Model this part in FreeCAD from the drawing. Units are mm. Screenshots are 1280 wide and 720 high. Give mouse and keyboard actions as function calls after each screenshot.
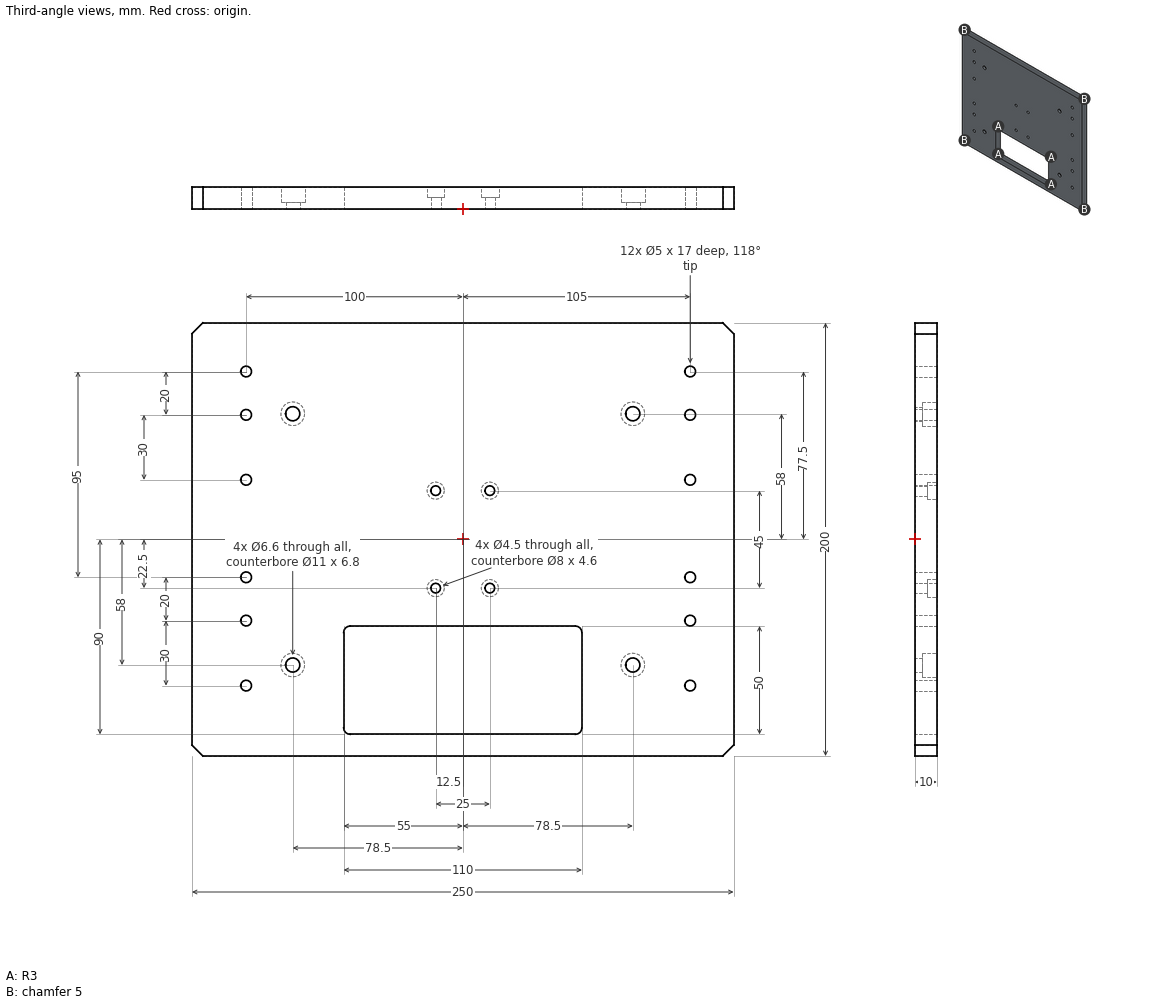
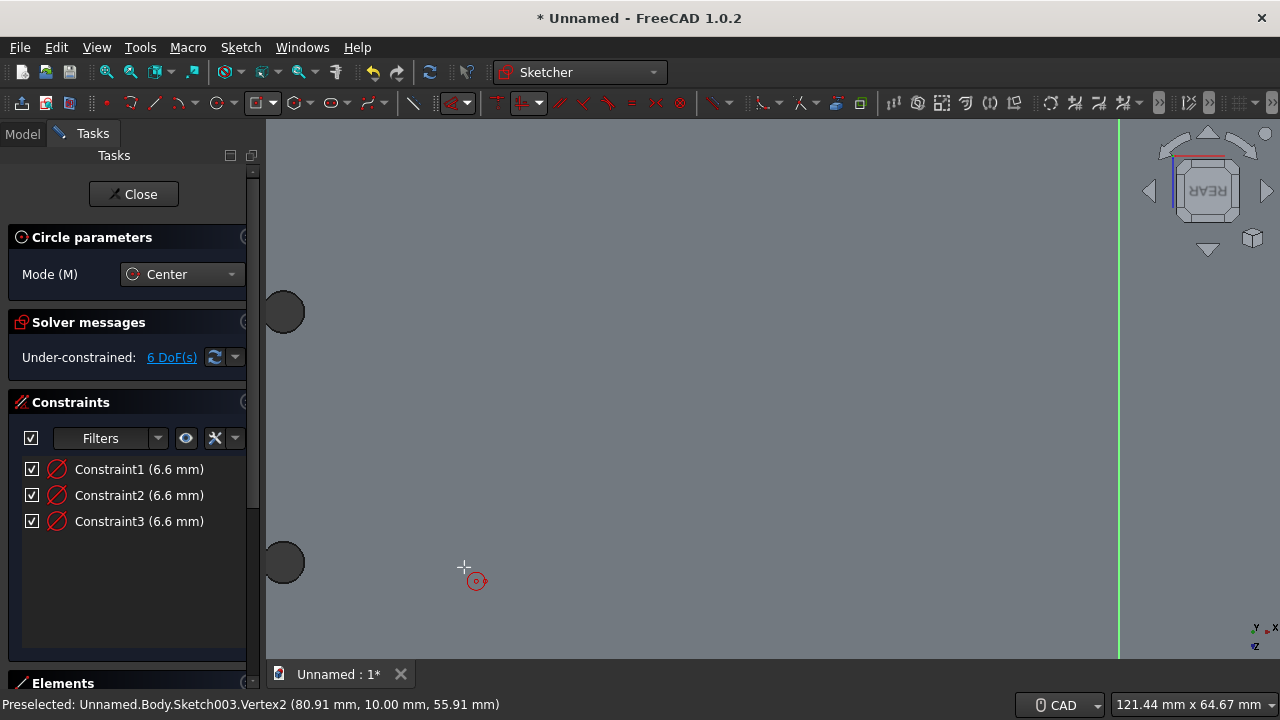
click(463, 567)
move(483, 547)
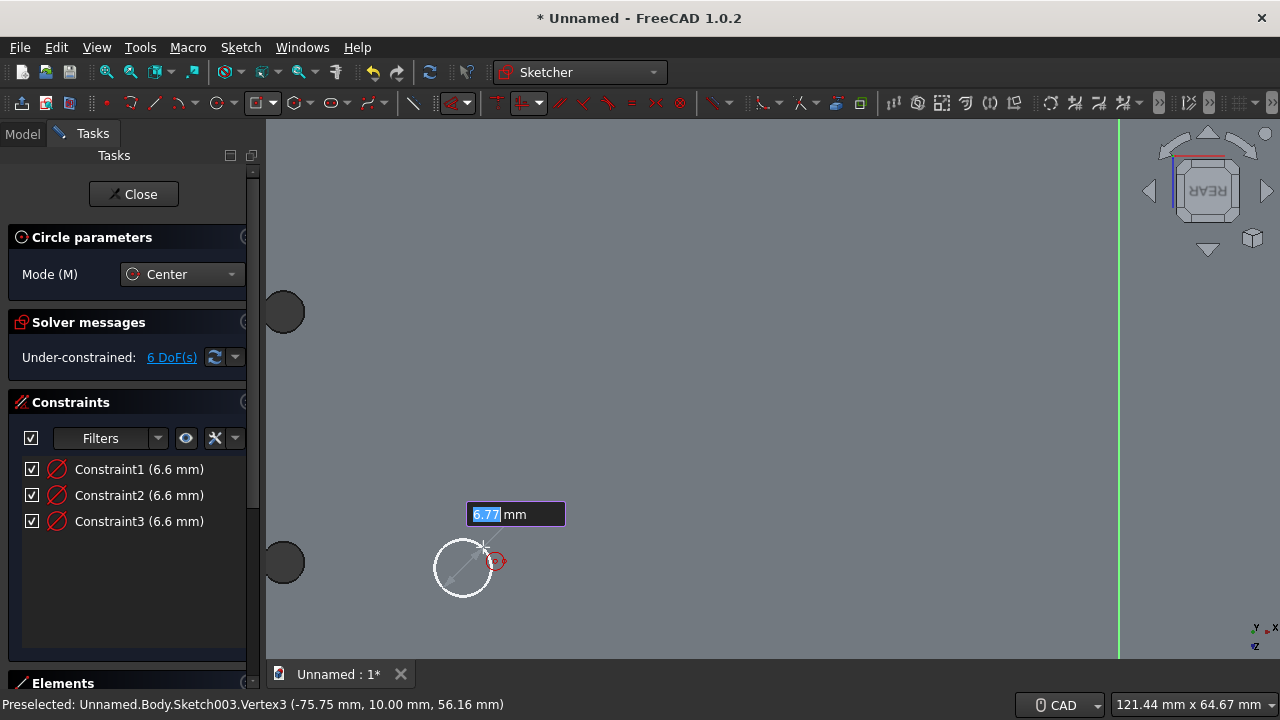
text(6.6)
key(Return)
key(Escape)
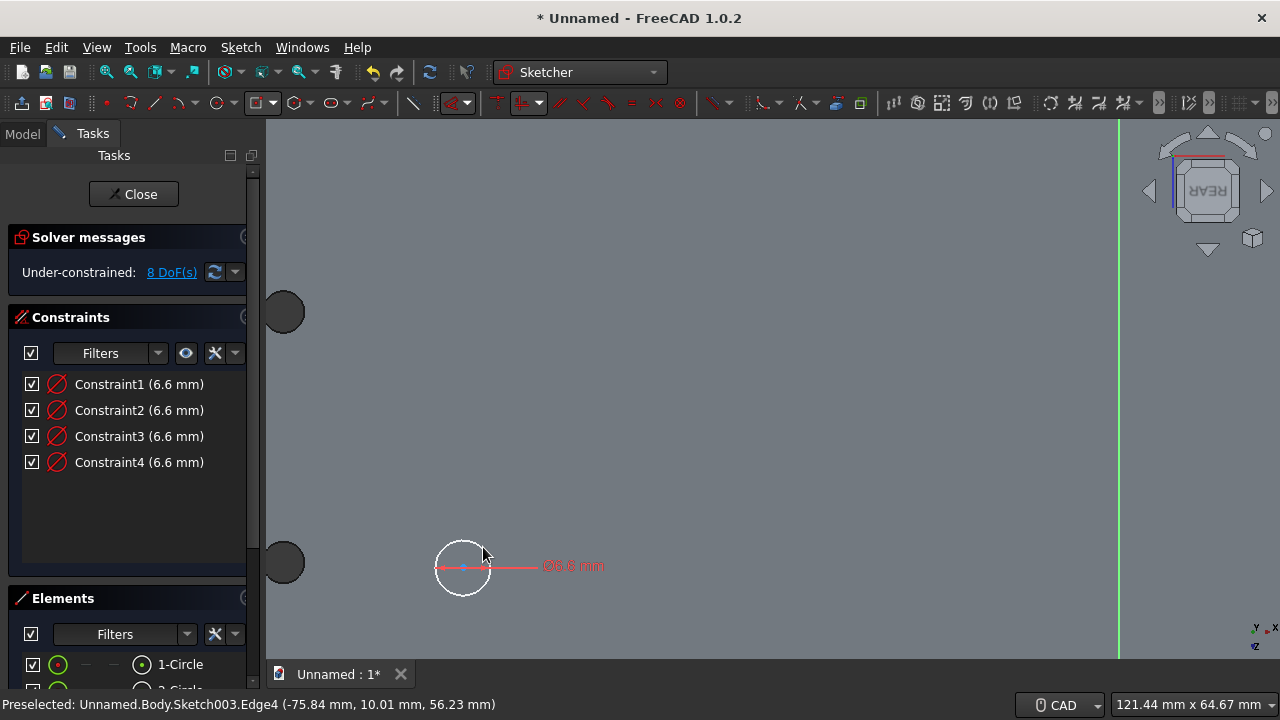
scroll(464, 567, down, 5)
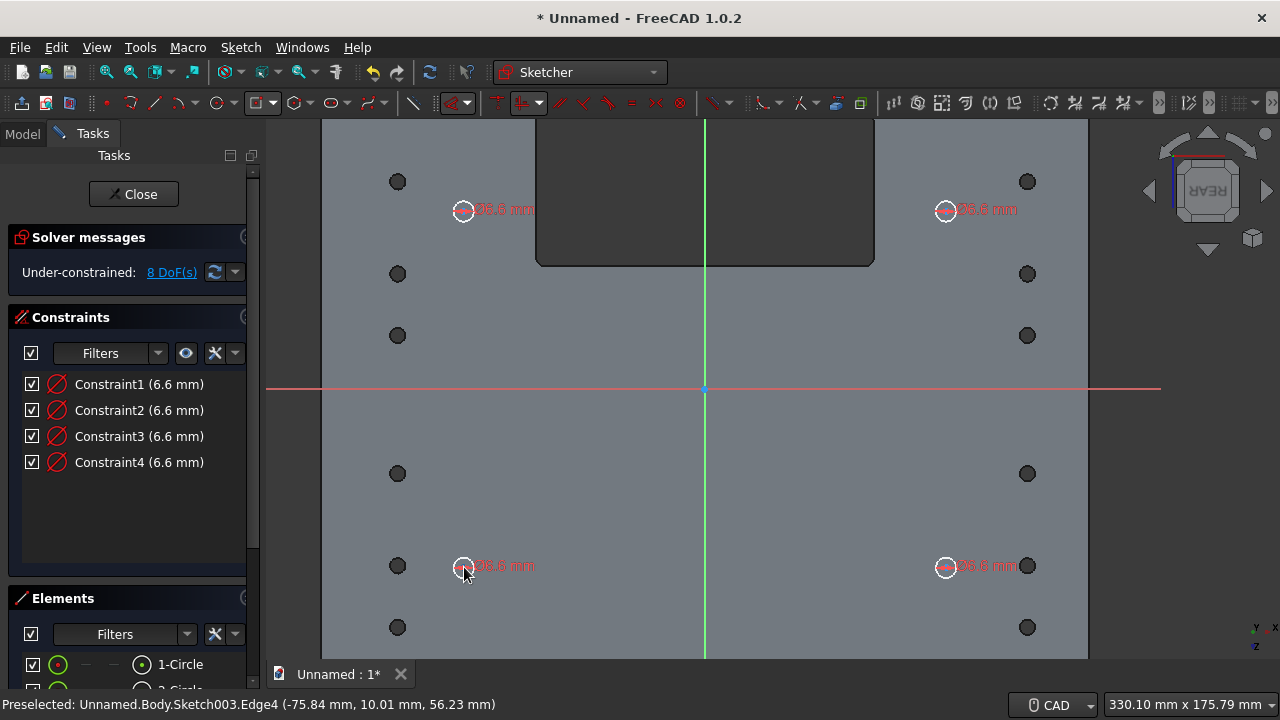
click(464, 211)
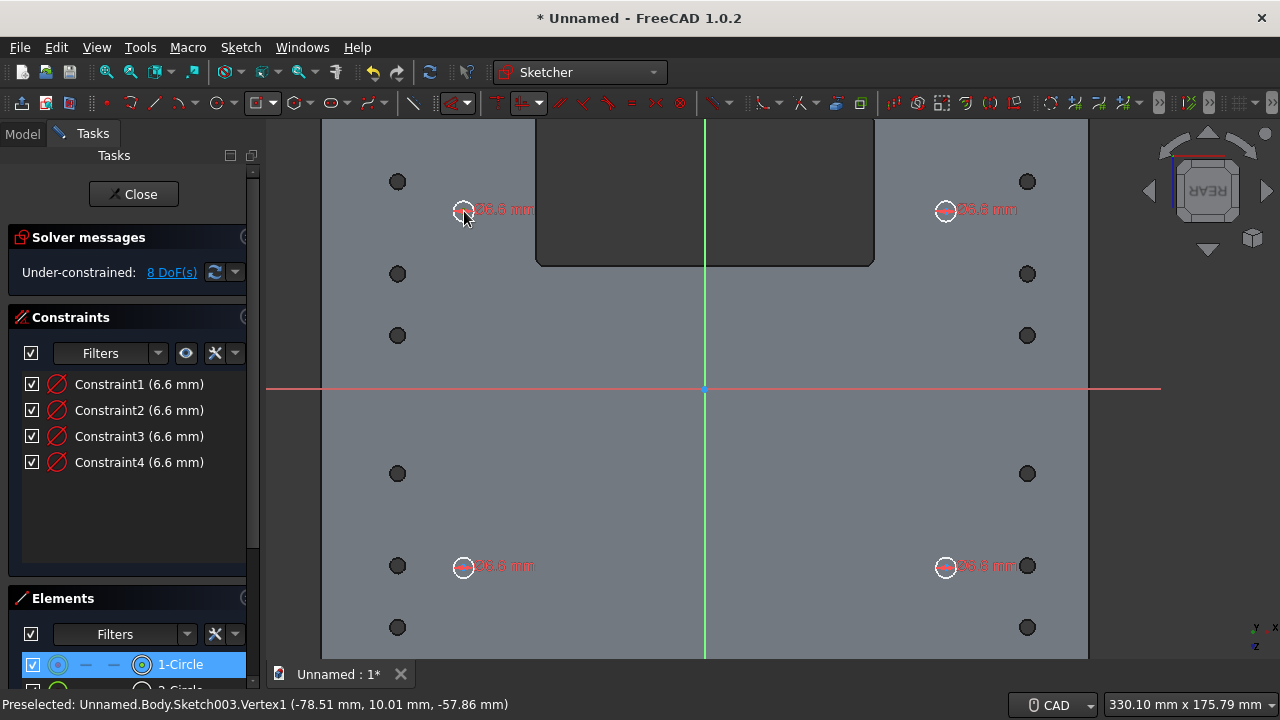
click(946, 211)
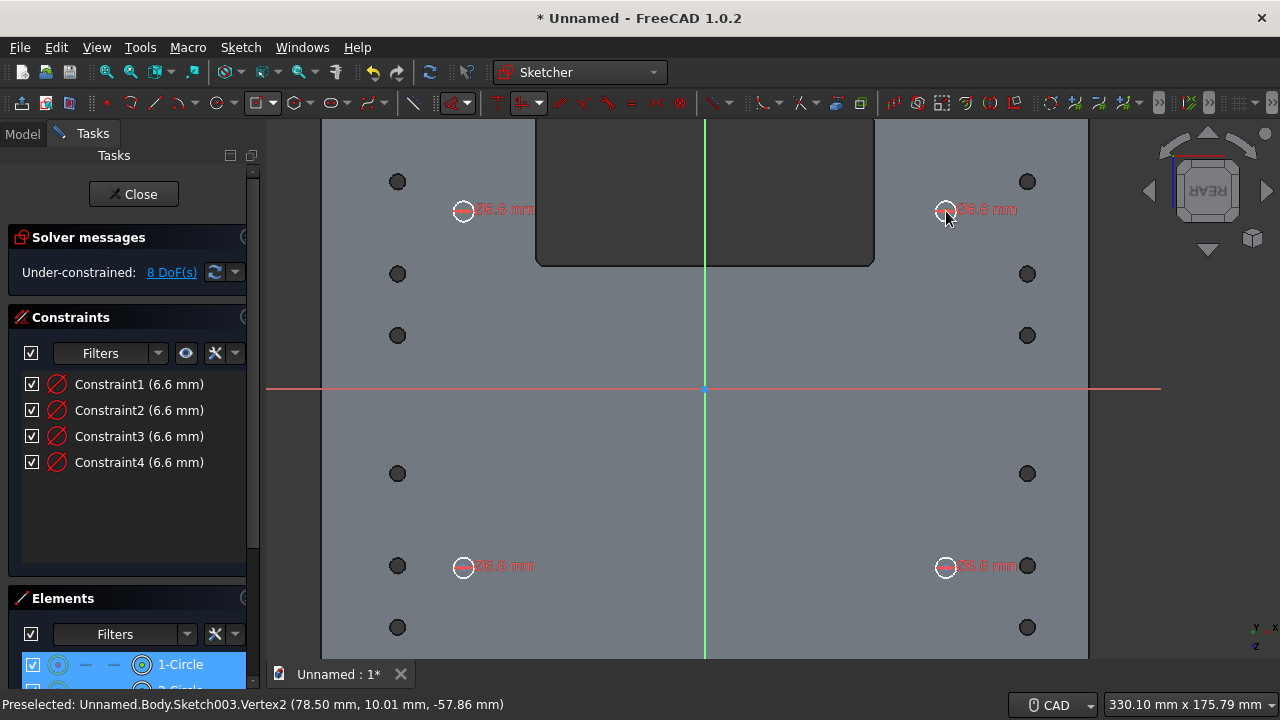
key(h)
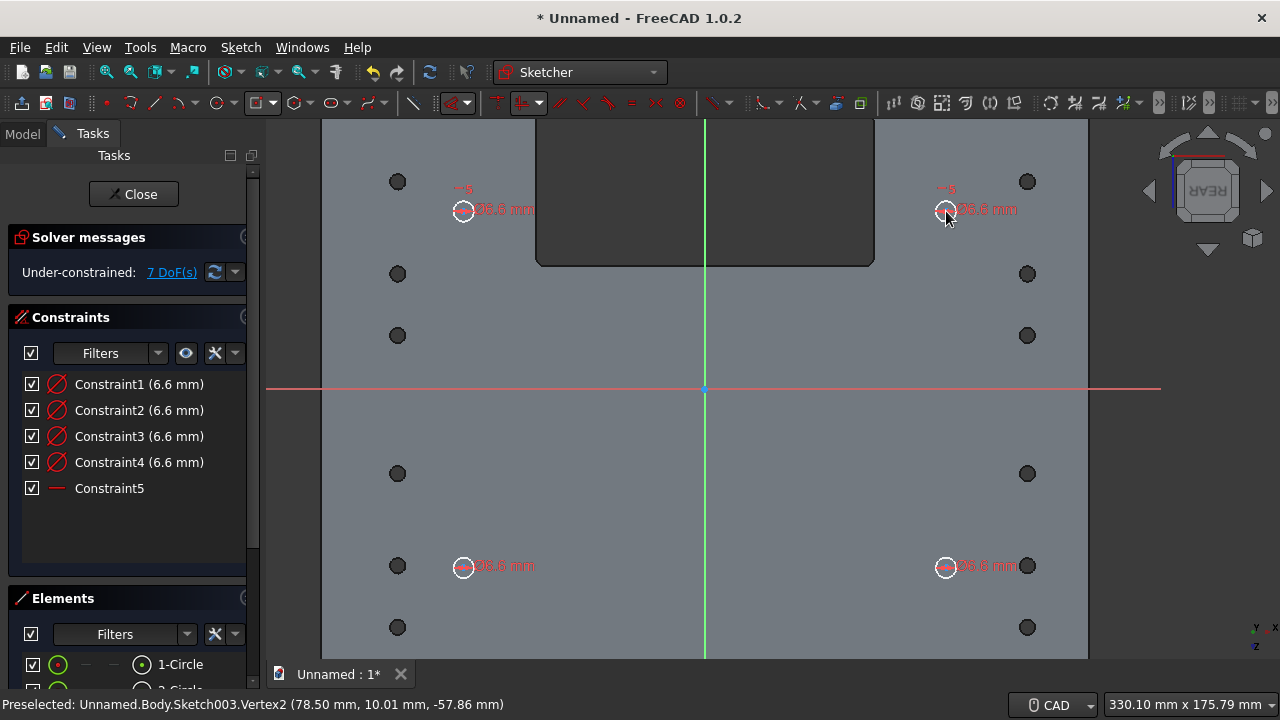
click(946, 211)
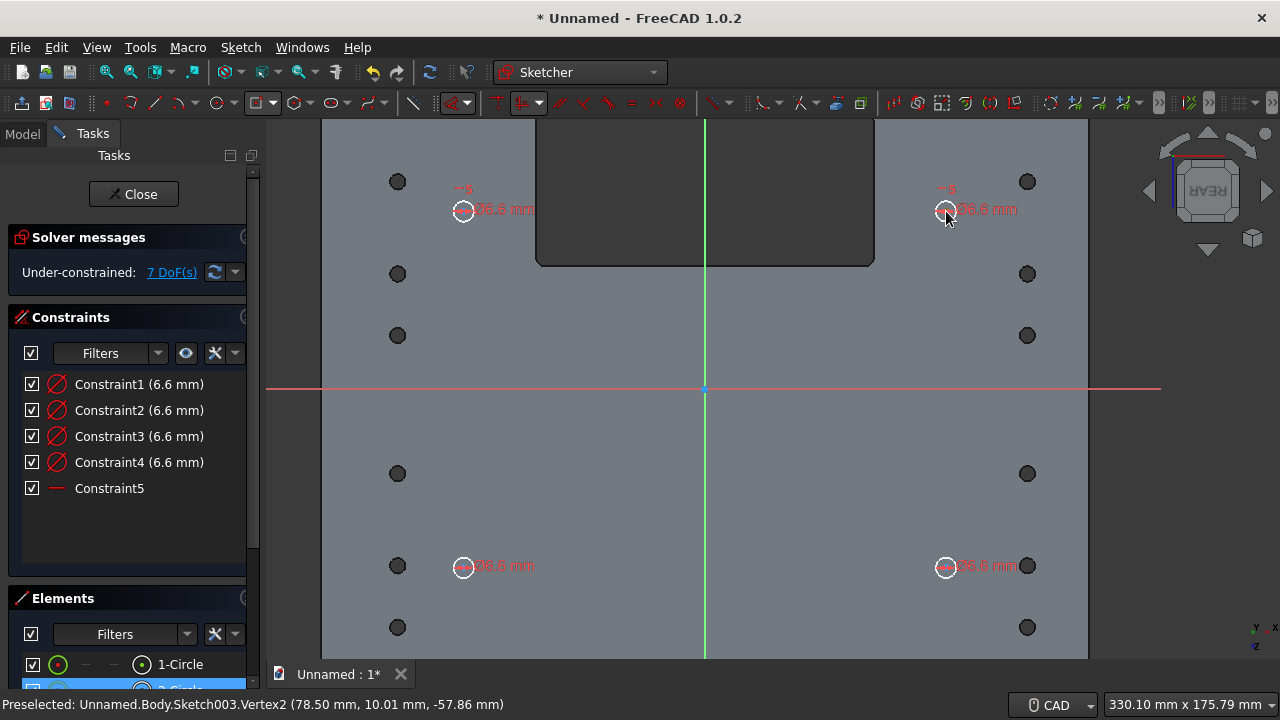
click(946, 568)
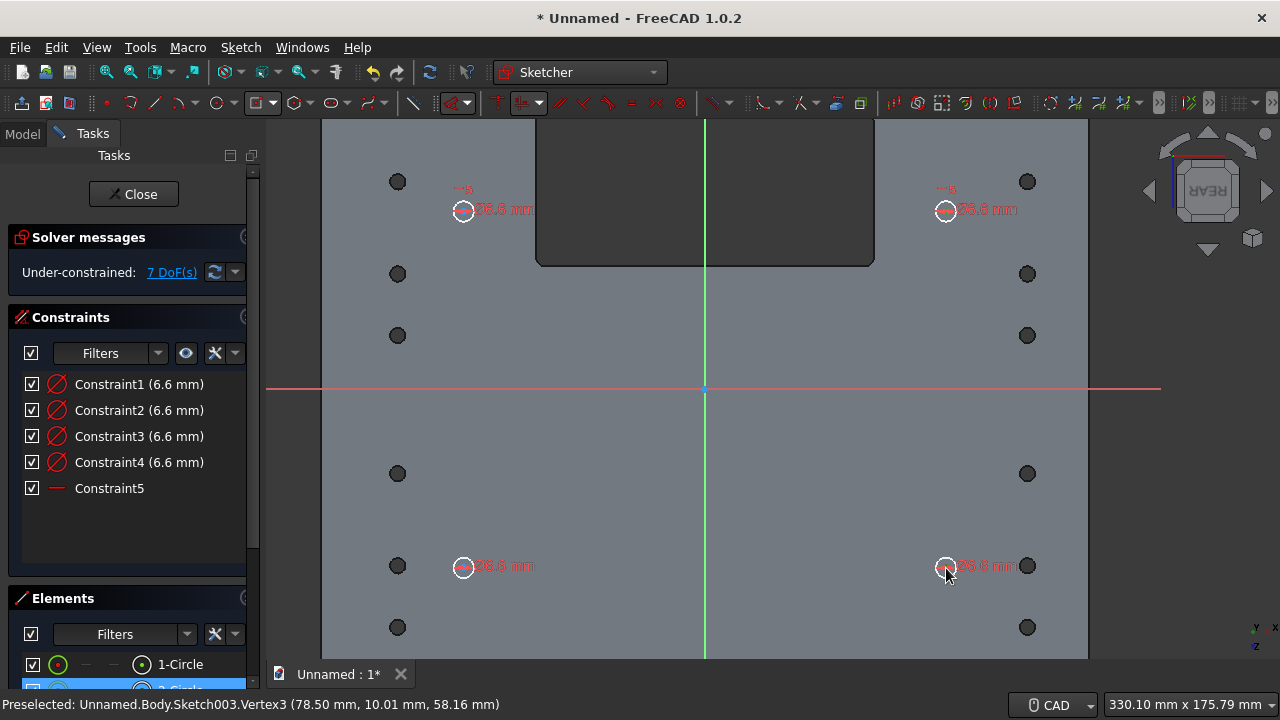
click(542, 104)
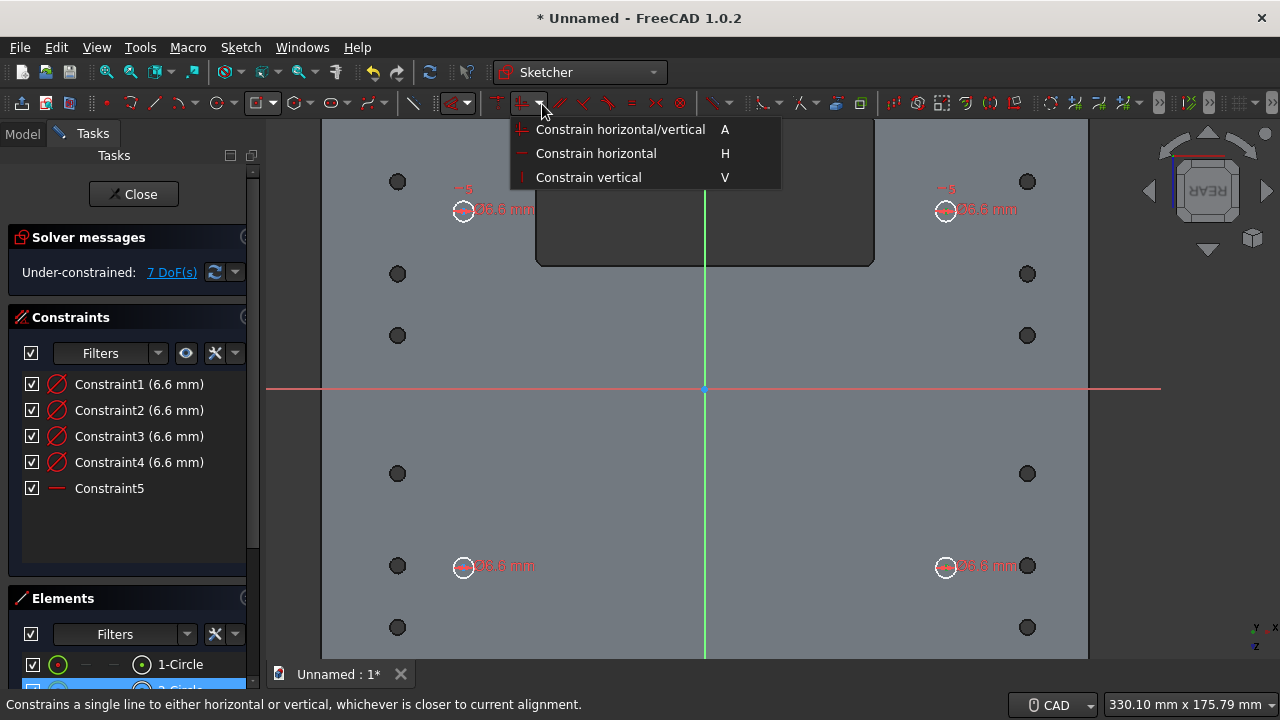
click(646, 177)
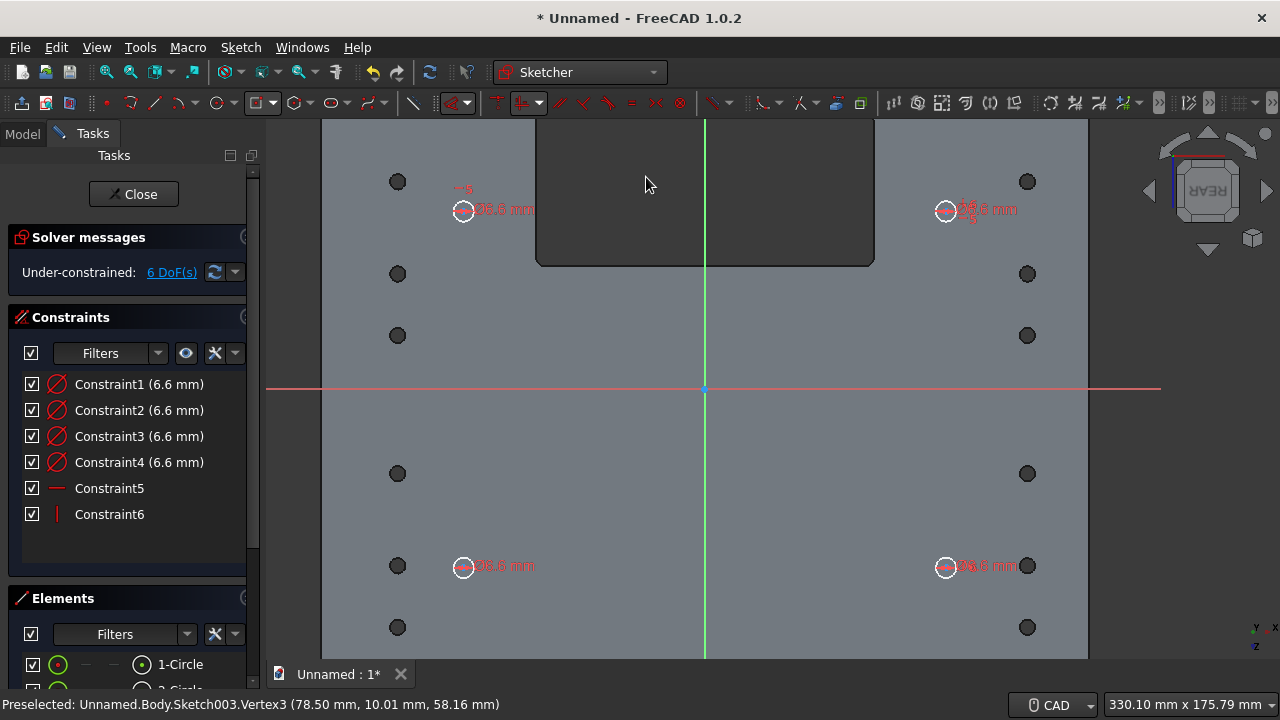
click(464, 211)